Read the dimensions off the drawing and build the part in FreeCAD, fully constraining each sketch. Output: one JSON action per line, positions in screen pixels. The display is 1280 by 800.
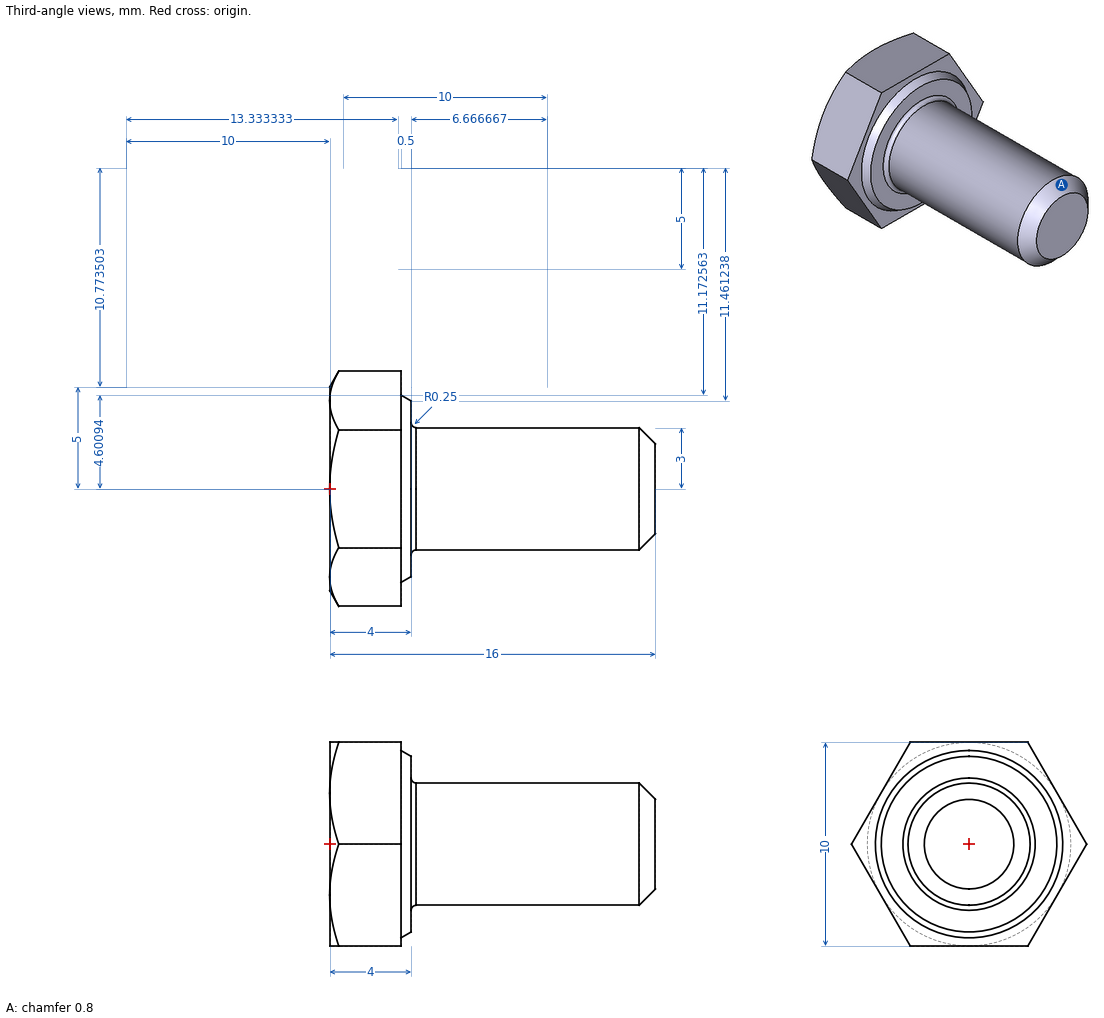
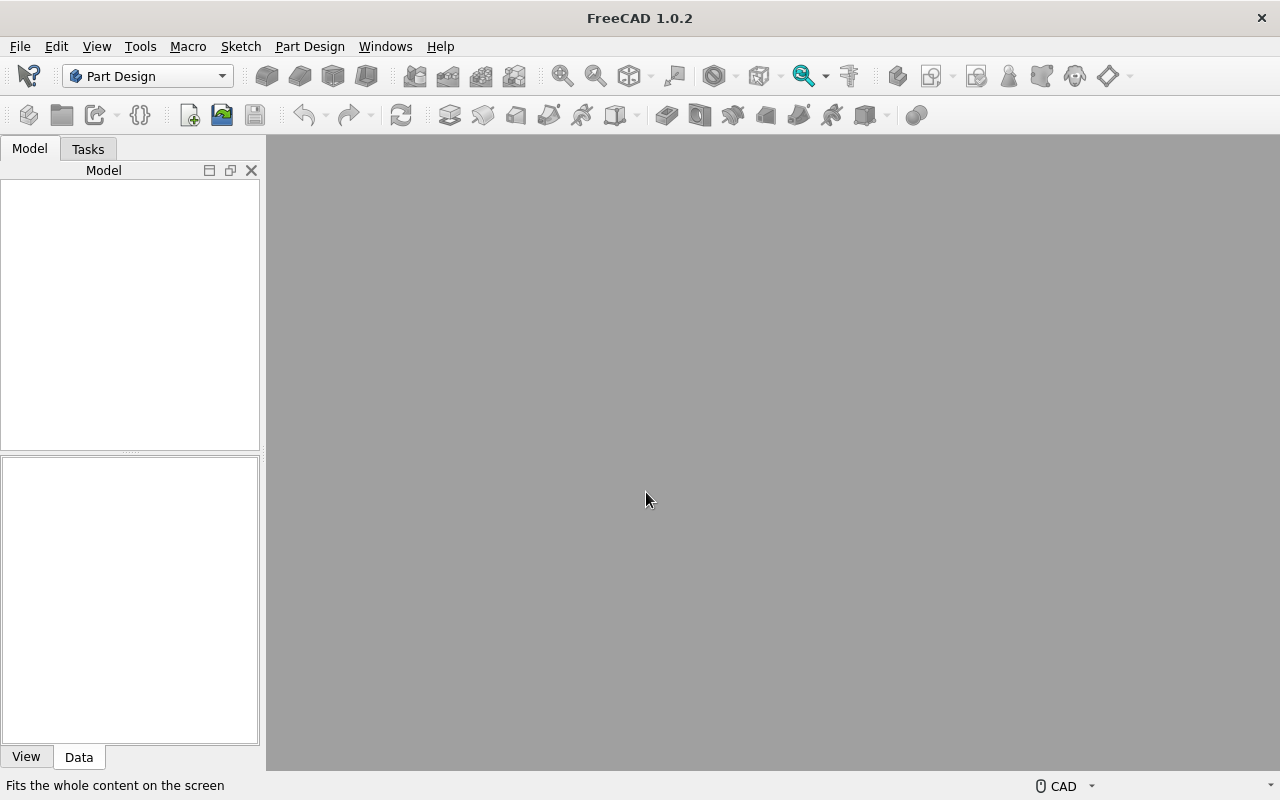
{"action": "left_click", "coordinate": [189, 116]}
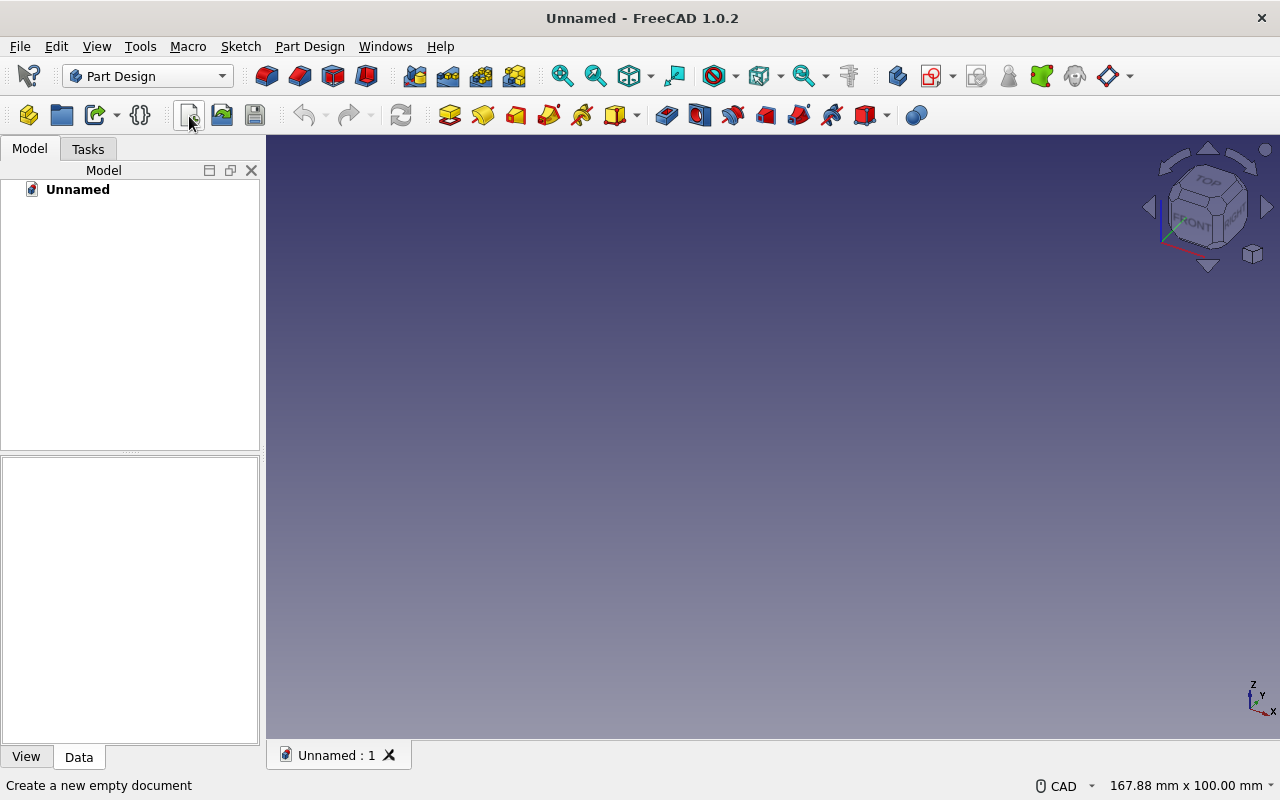
{"action": "left_click", "coordinate": [930, 76]}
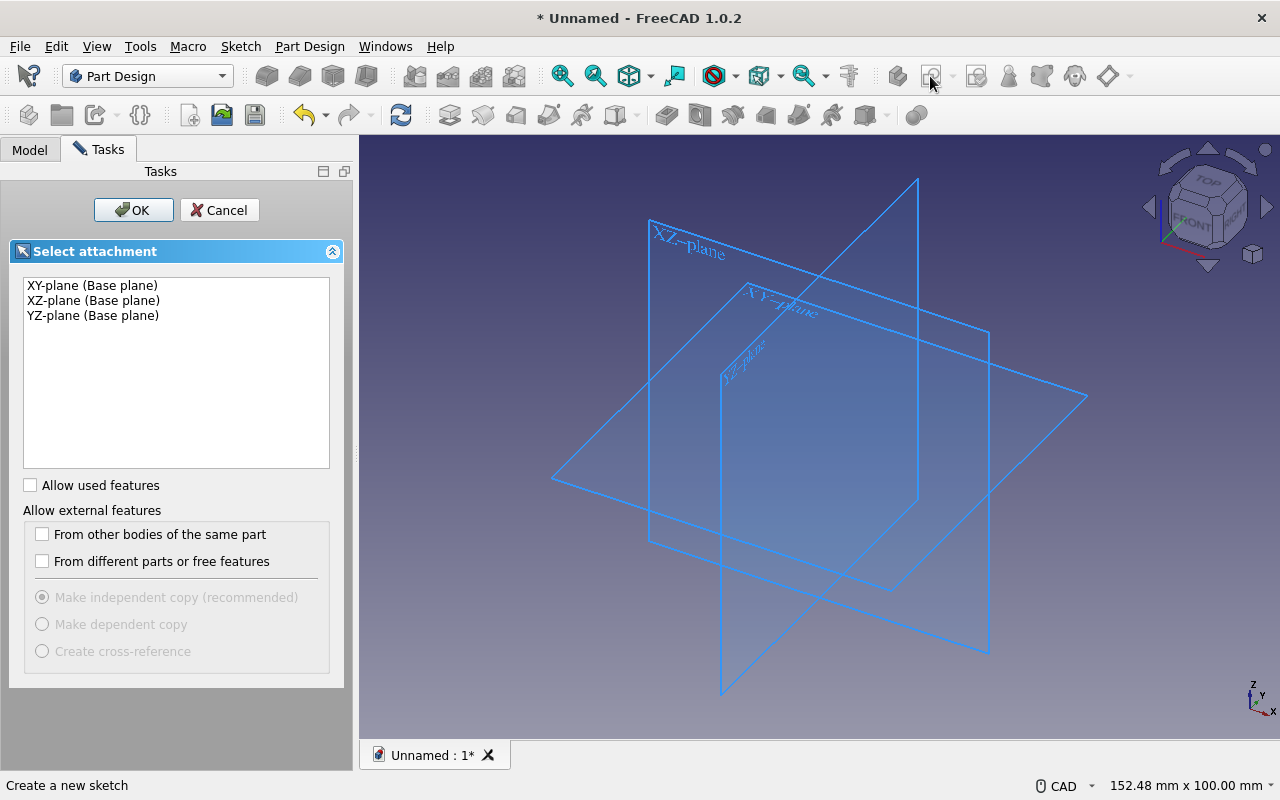
{"action": "left_click", "coordinate": [84, 316]}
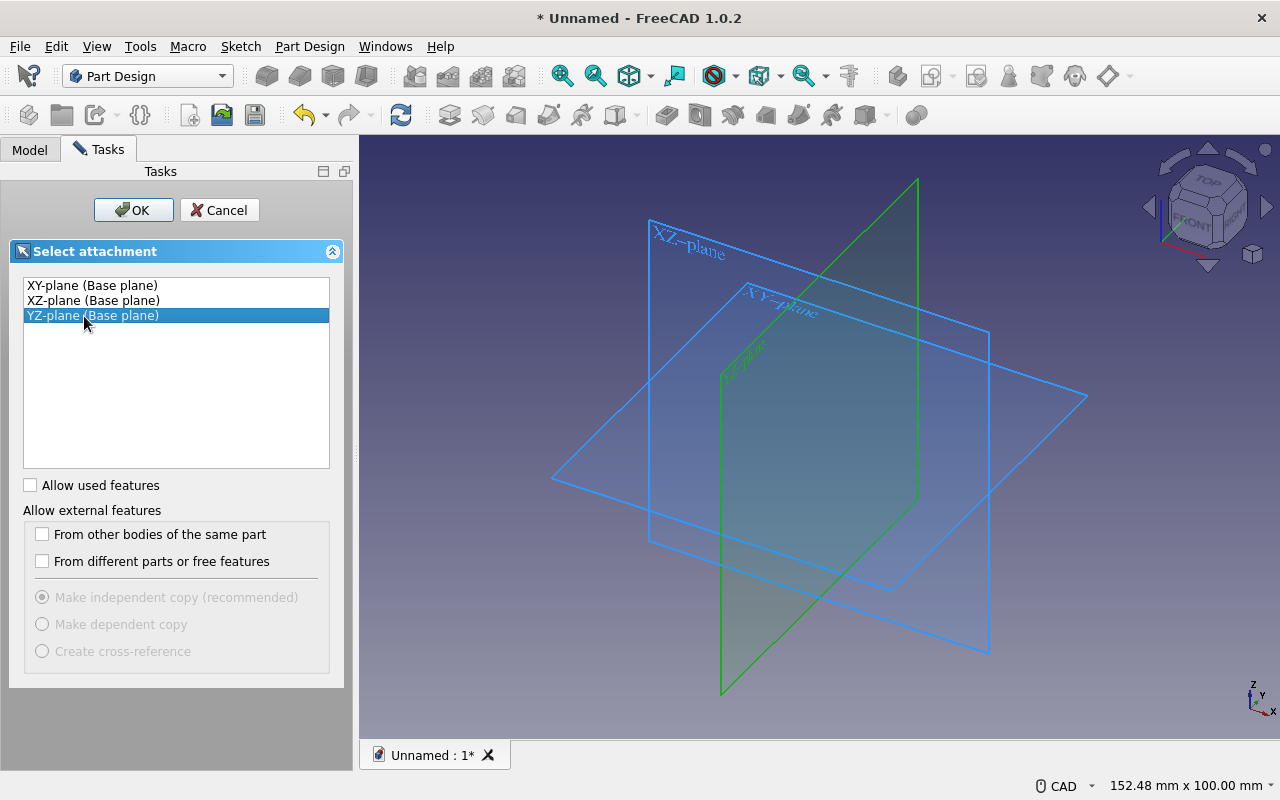
{"action": "left_click", "coordinate": [134, 210]}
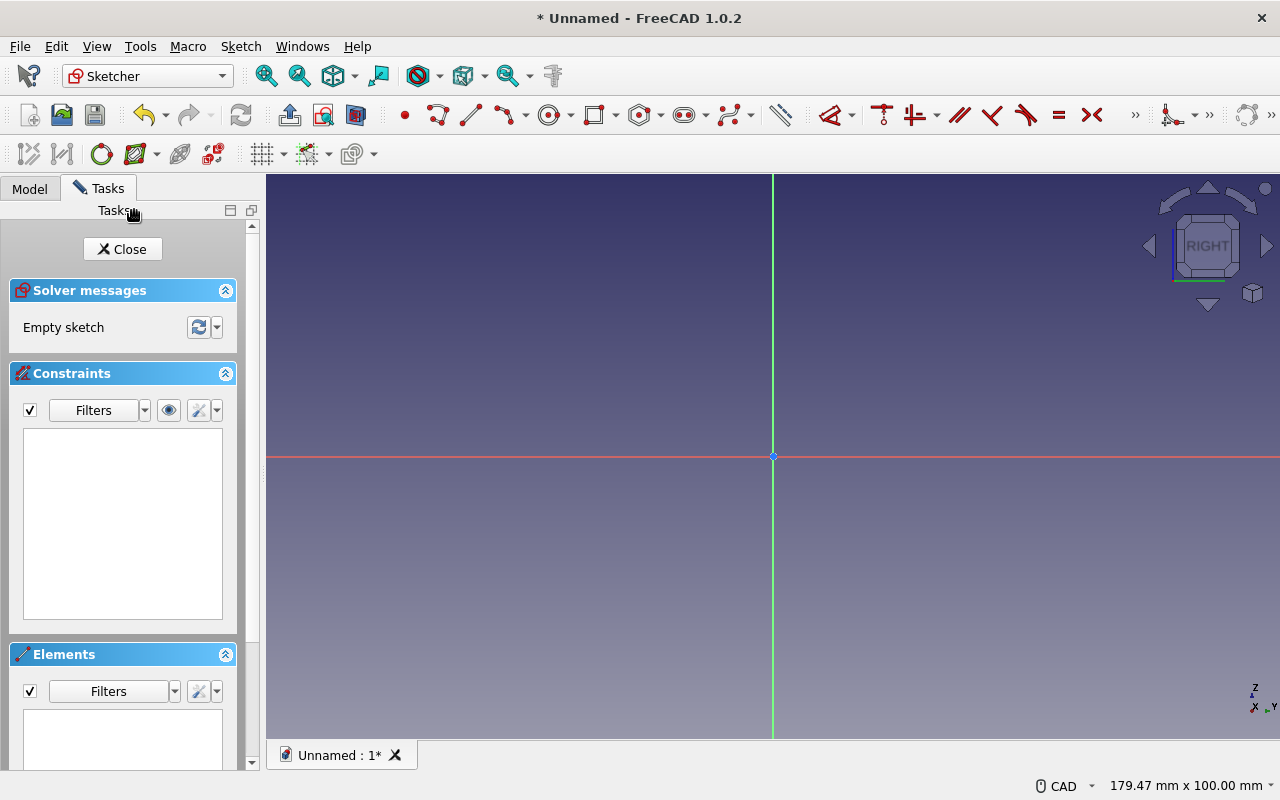
{"action": "scroll", "coordinate": [787, 456], "scroll_direction": "up", "scroll_amount": 9}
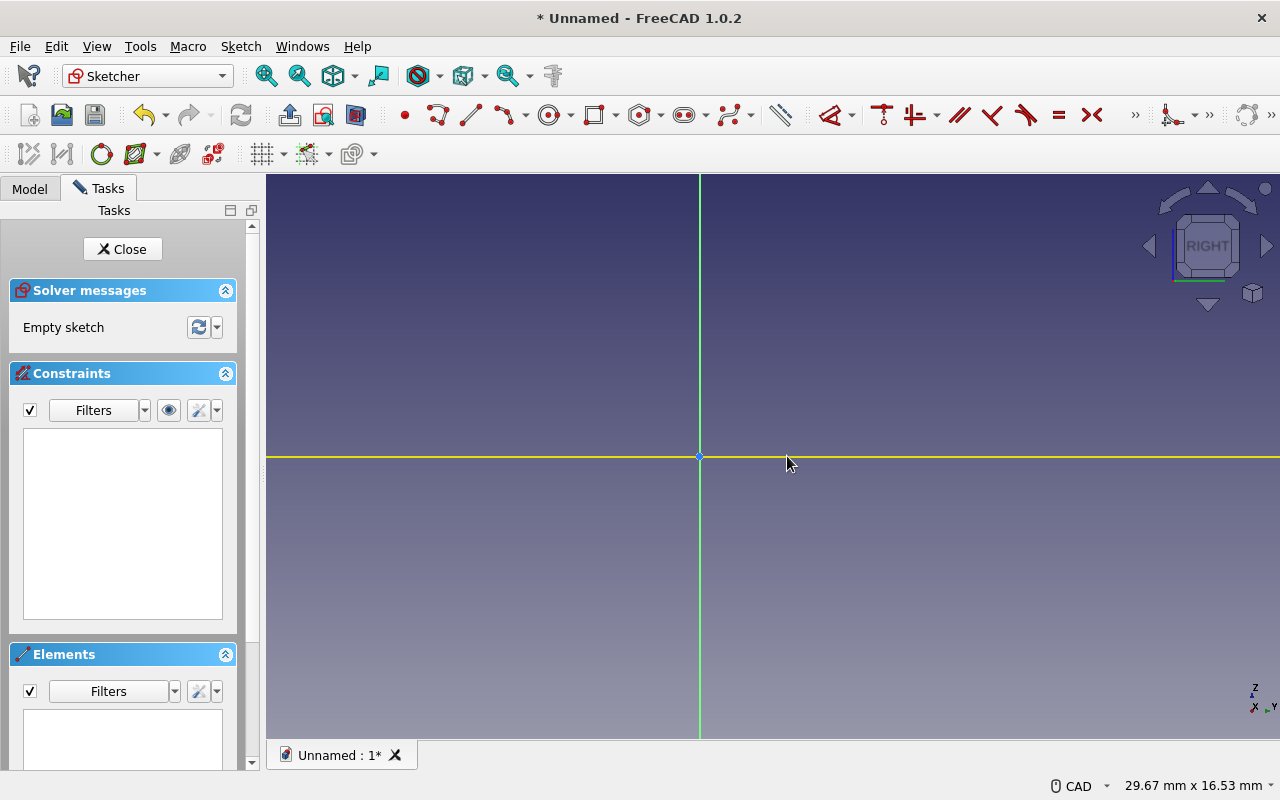
{"action": "left_click", "coordinate": [638, 116]}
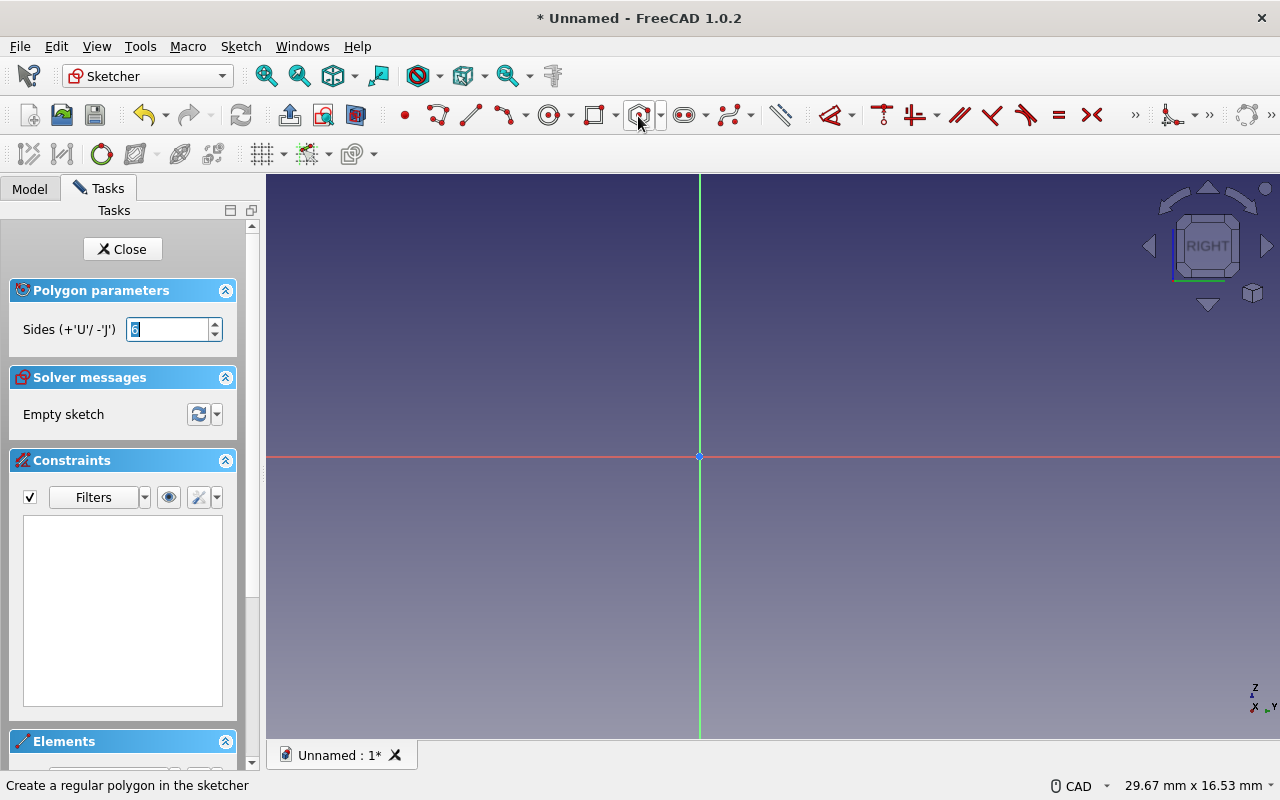
{"action": "left_click", "coordinate": [700, 456]}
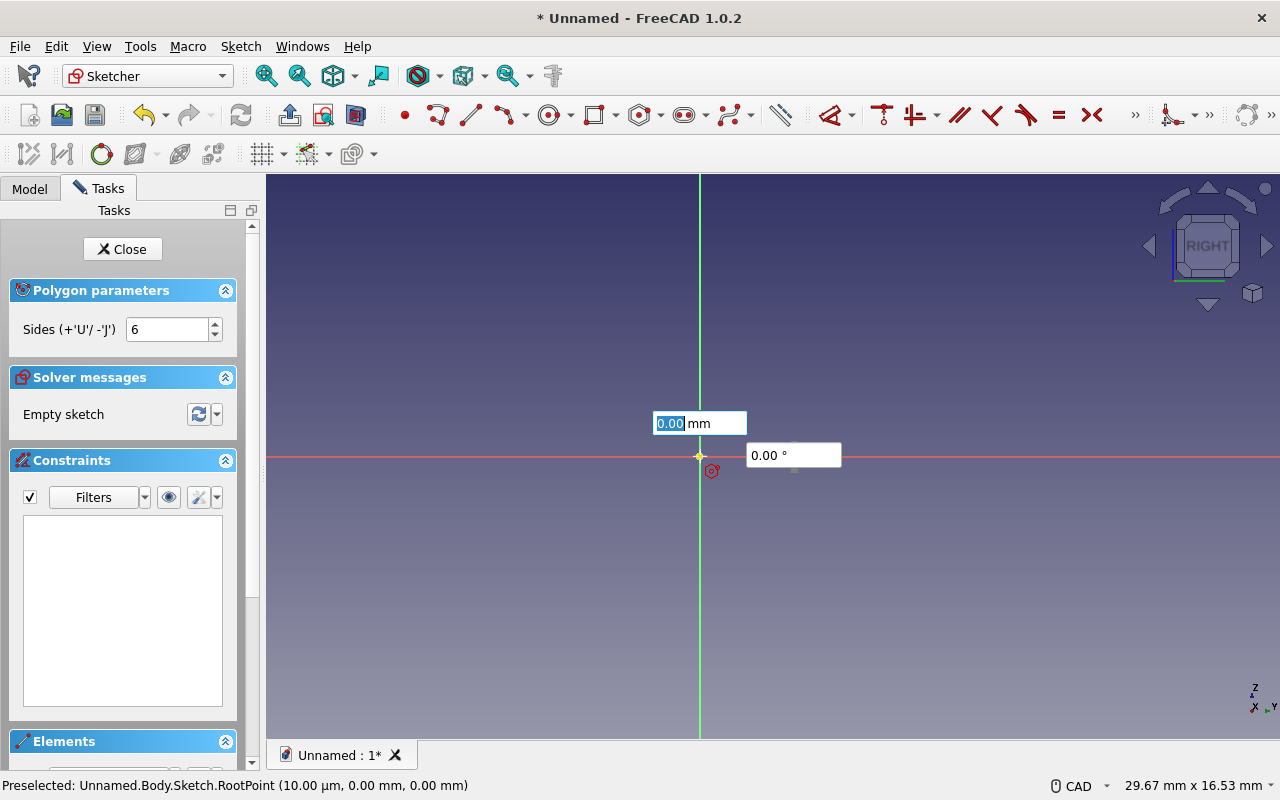
{"action": "left_click", "coordinate": [897, 456]}
{"action": "right_click", "coordinate": [897, 456]}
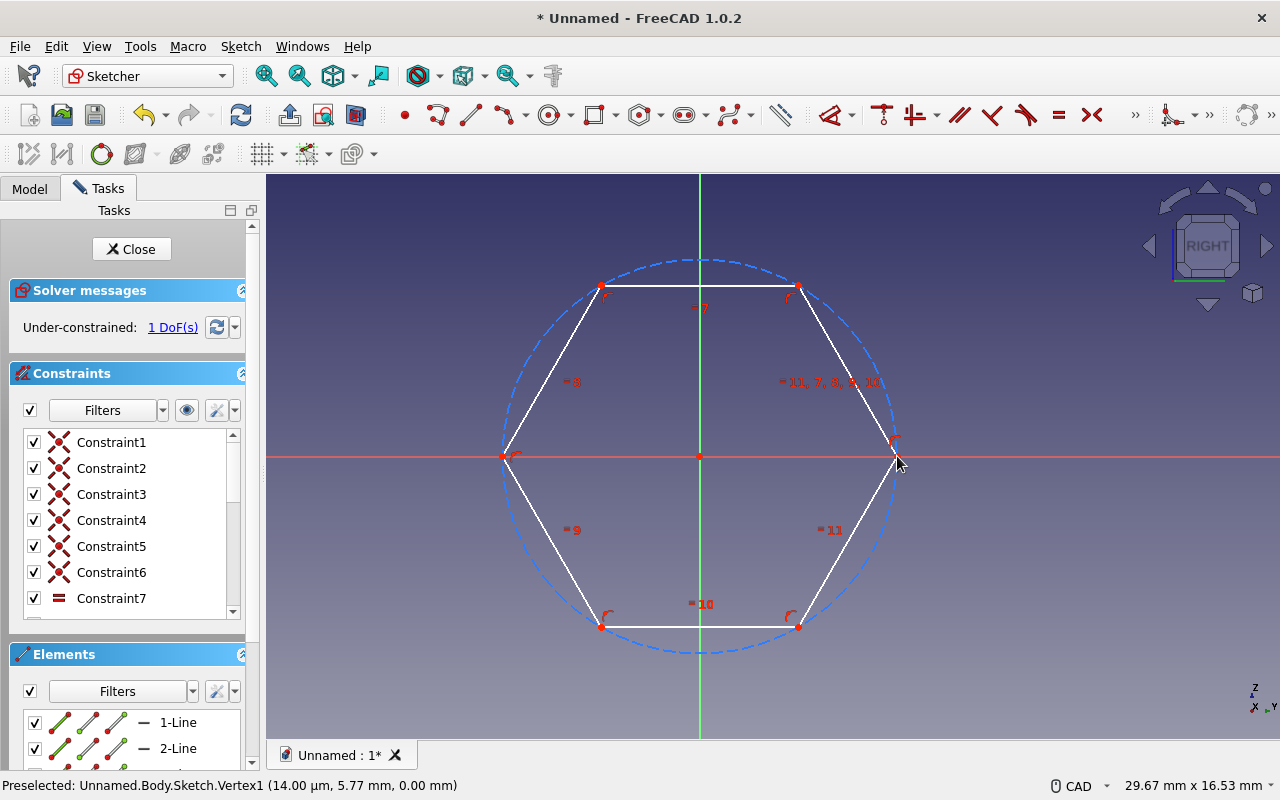
{"action": "left_click", "coordinate": [601, 627]}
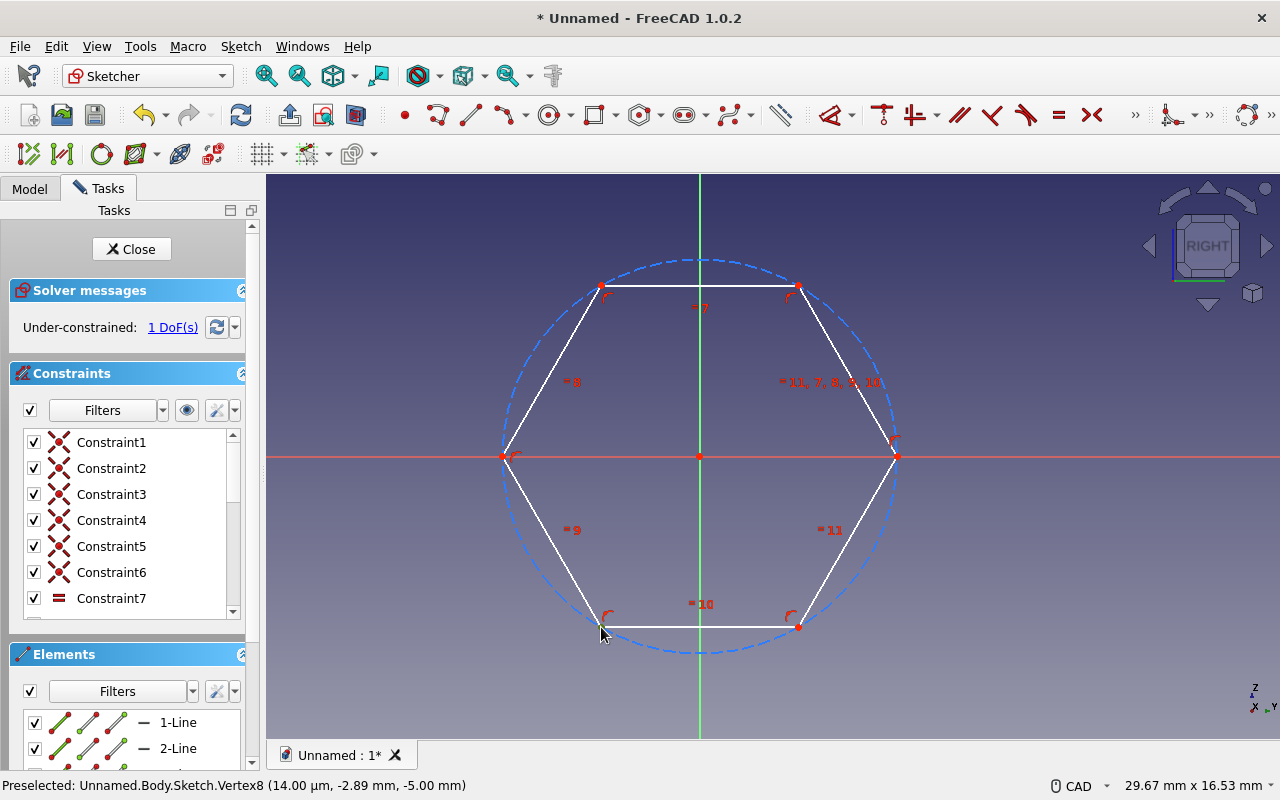
{"action": "left_click", "coordinate": [798, 286]}